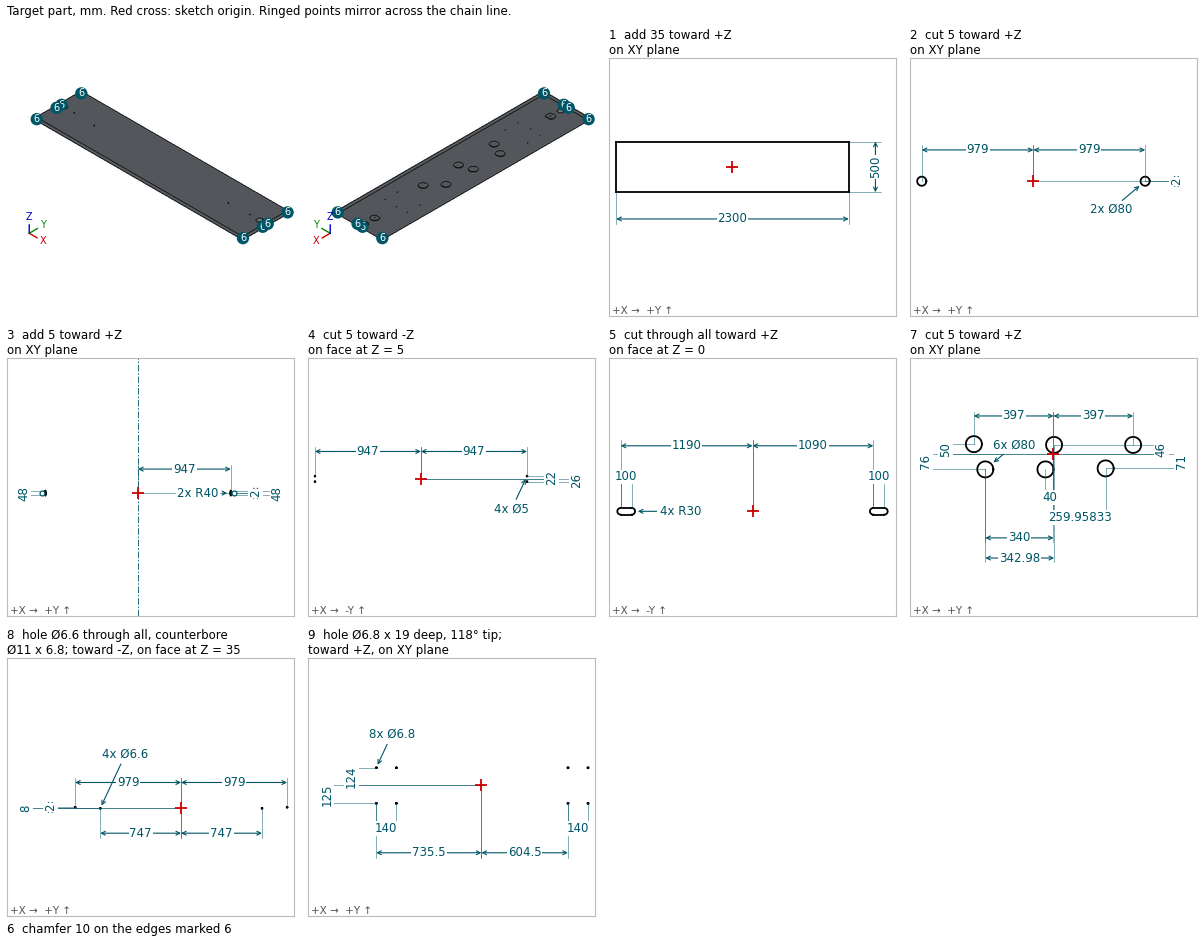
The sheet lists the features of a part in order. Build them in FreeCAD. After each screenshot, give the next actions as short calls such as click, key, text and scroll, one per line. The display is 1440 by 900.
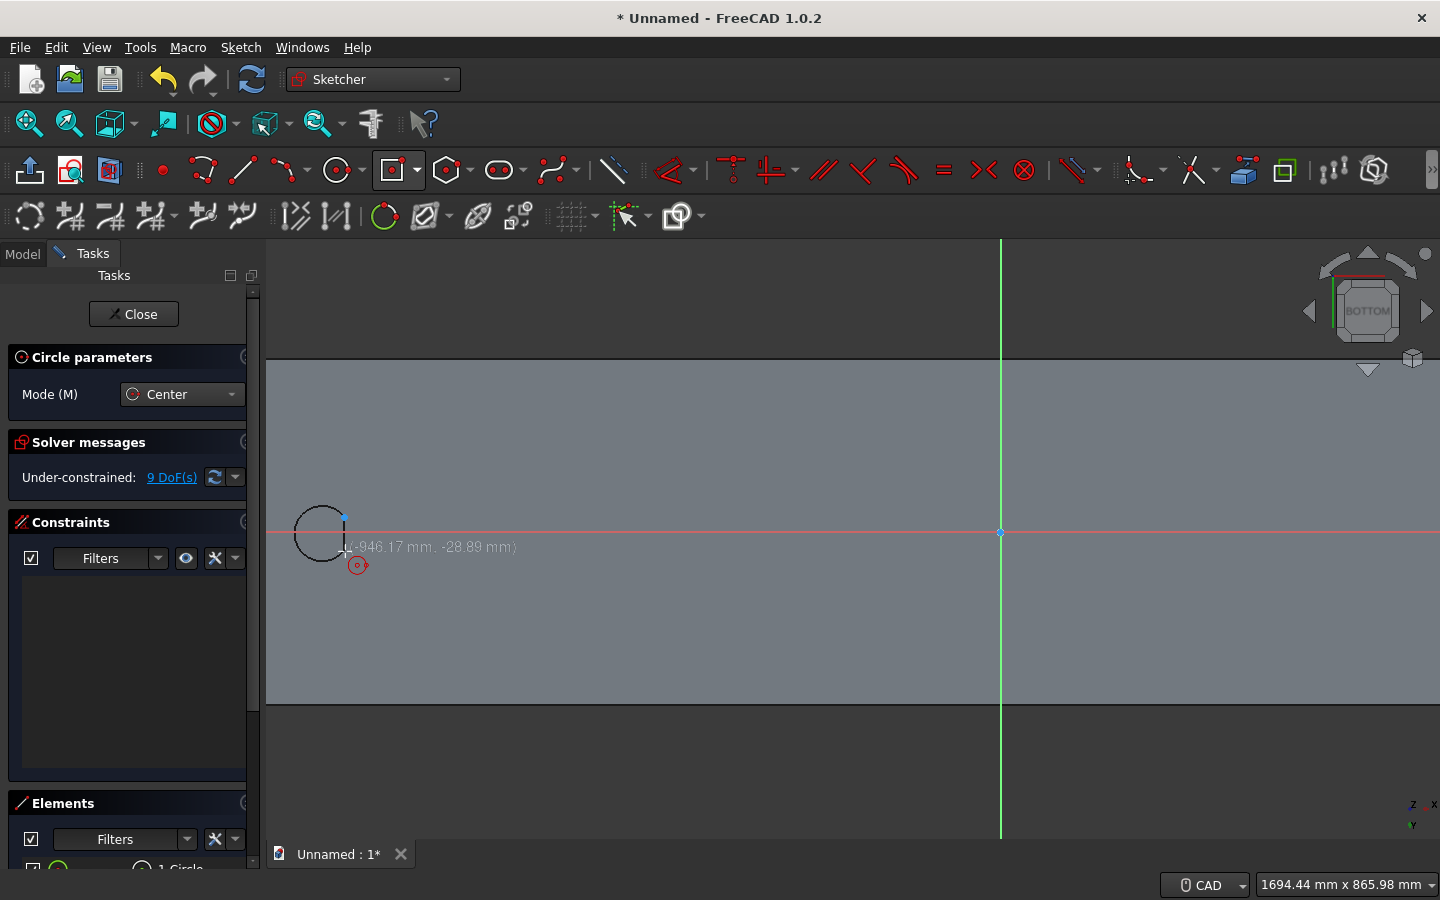
click(344, 550)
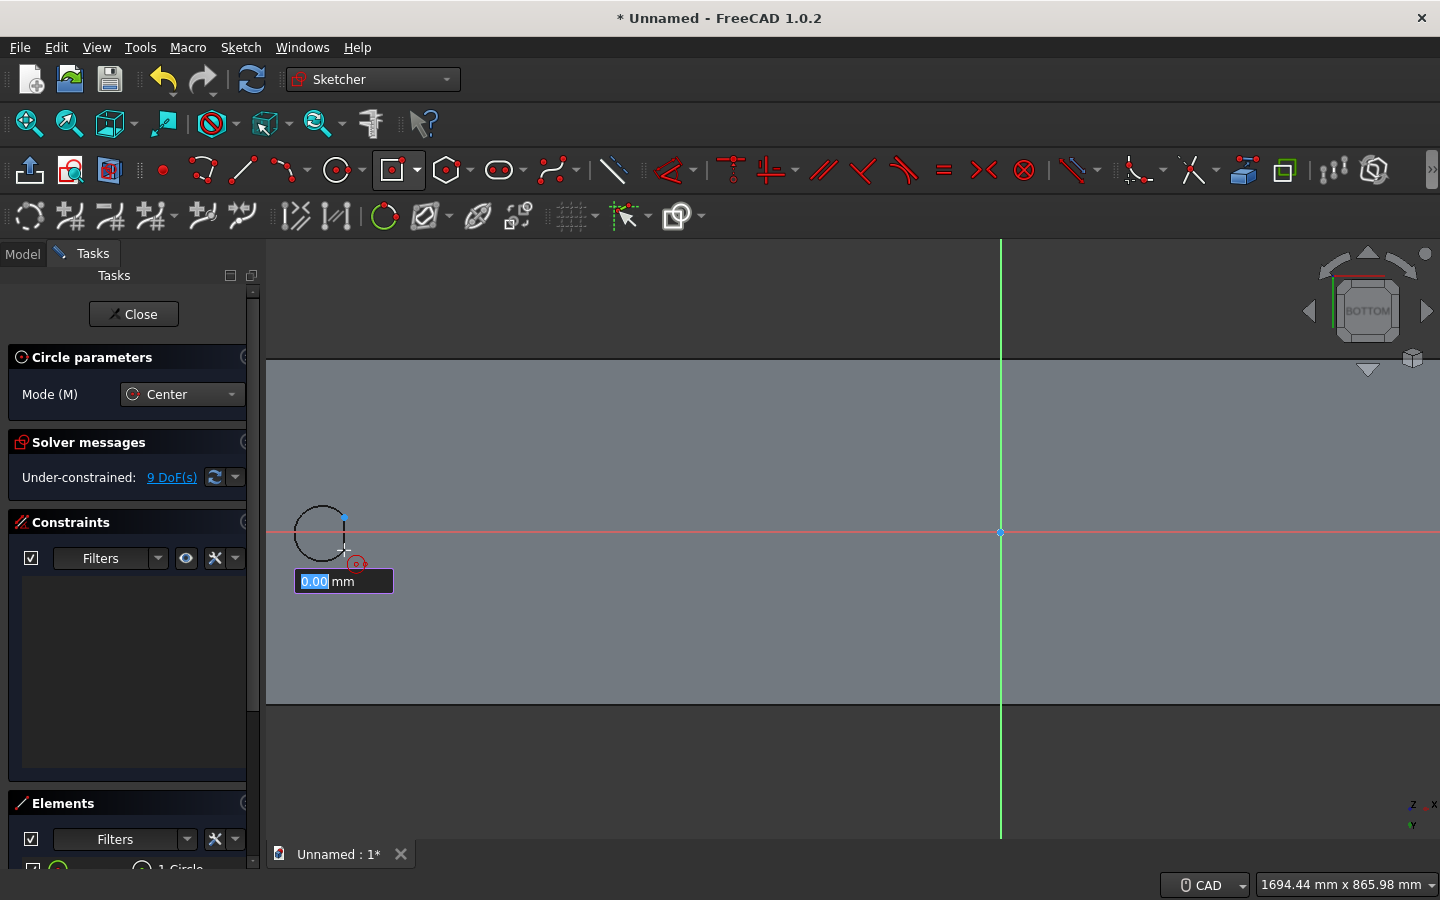
scroll(346, 549, up, 12)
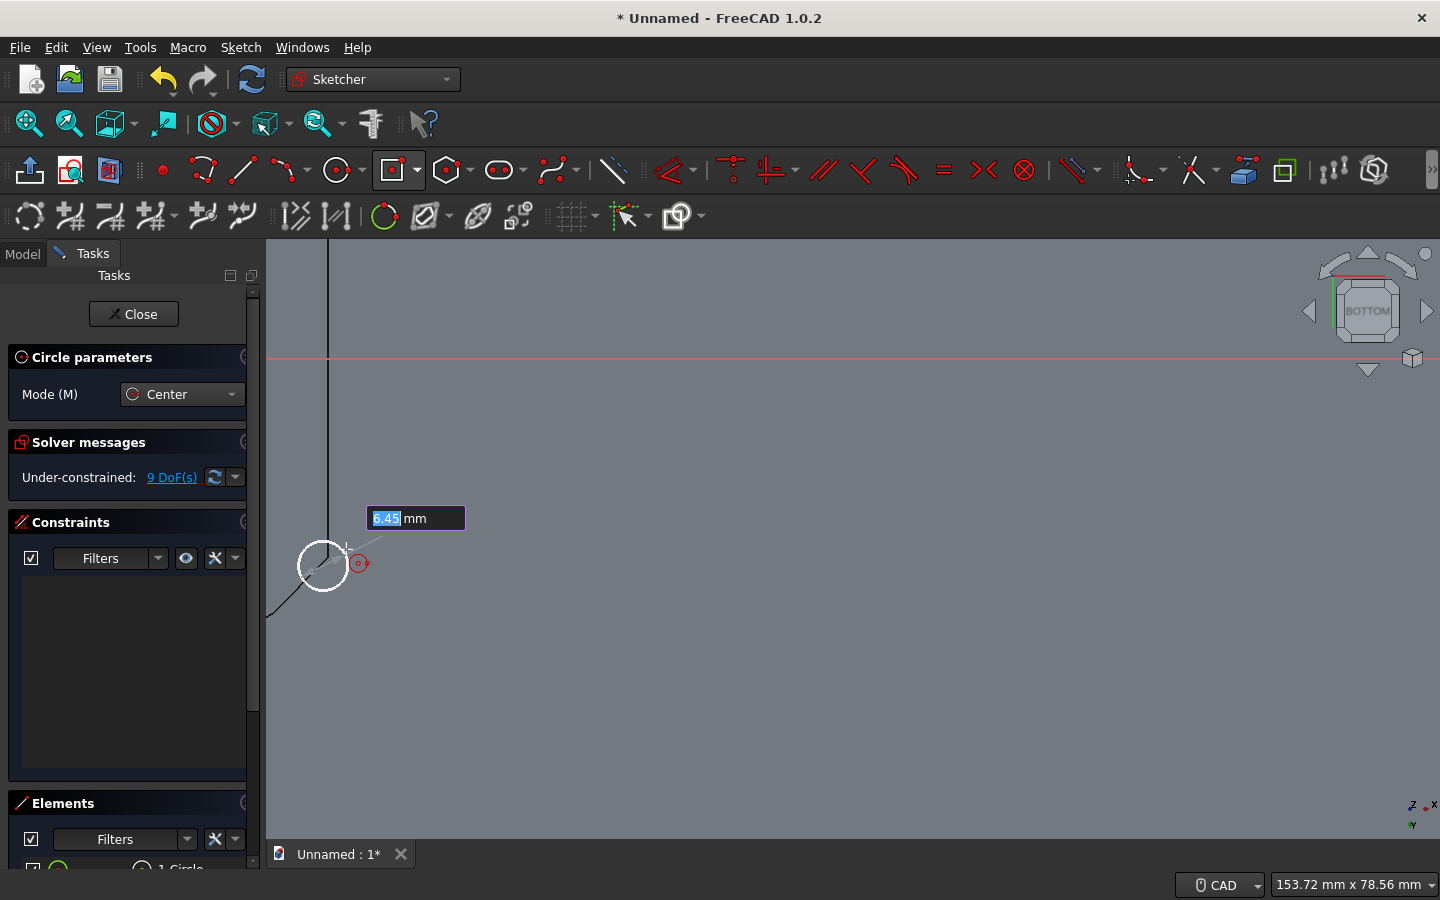
click(341, 544)
key(Escape)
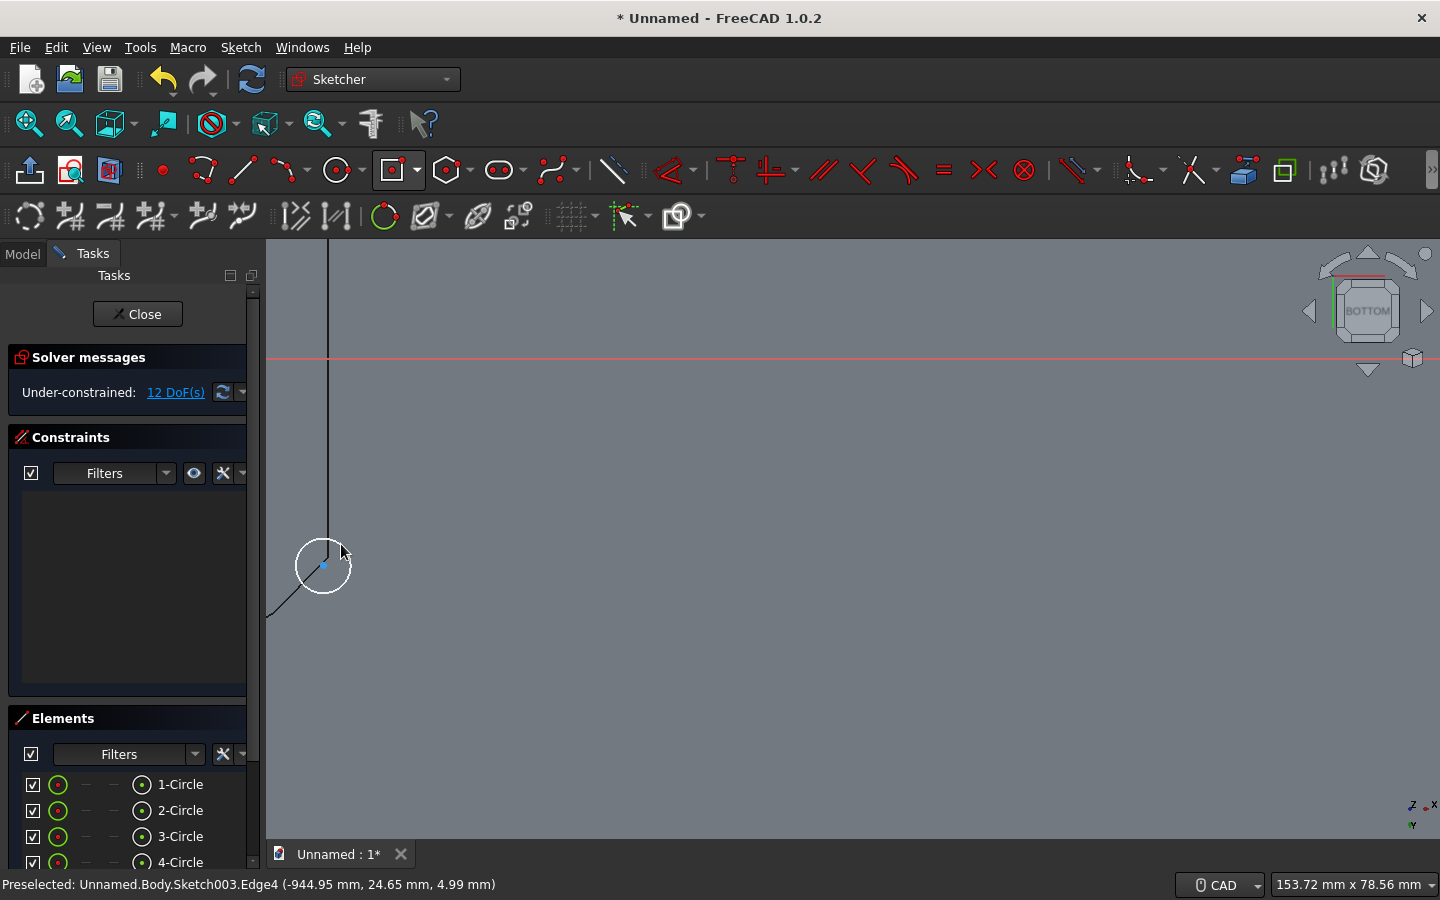
scroll(429, 548, down, 15)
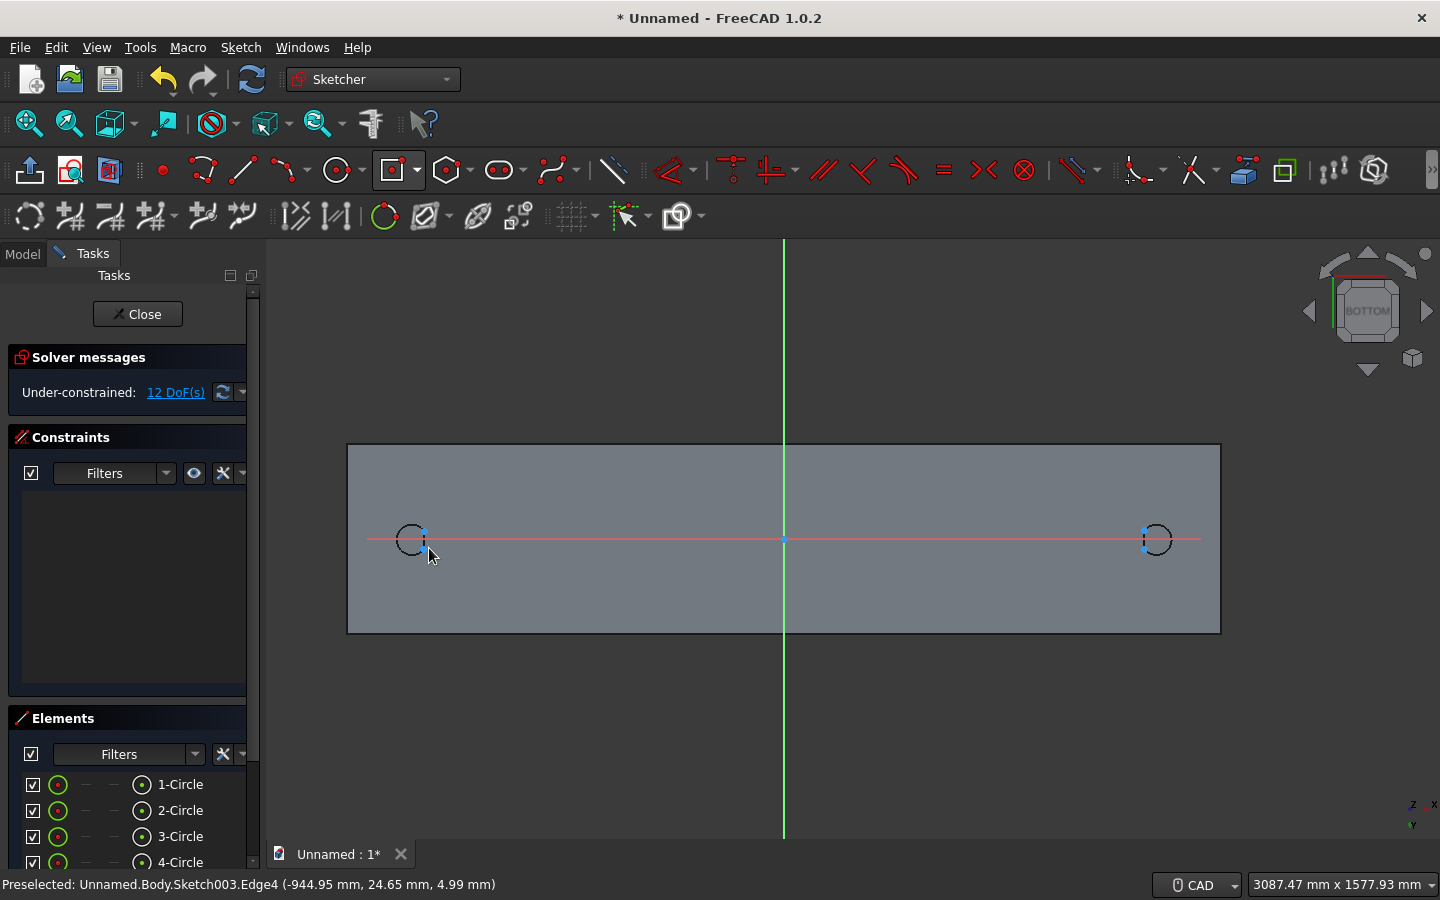
scroll(1145, 530, up, 13)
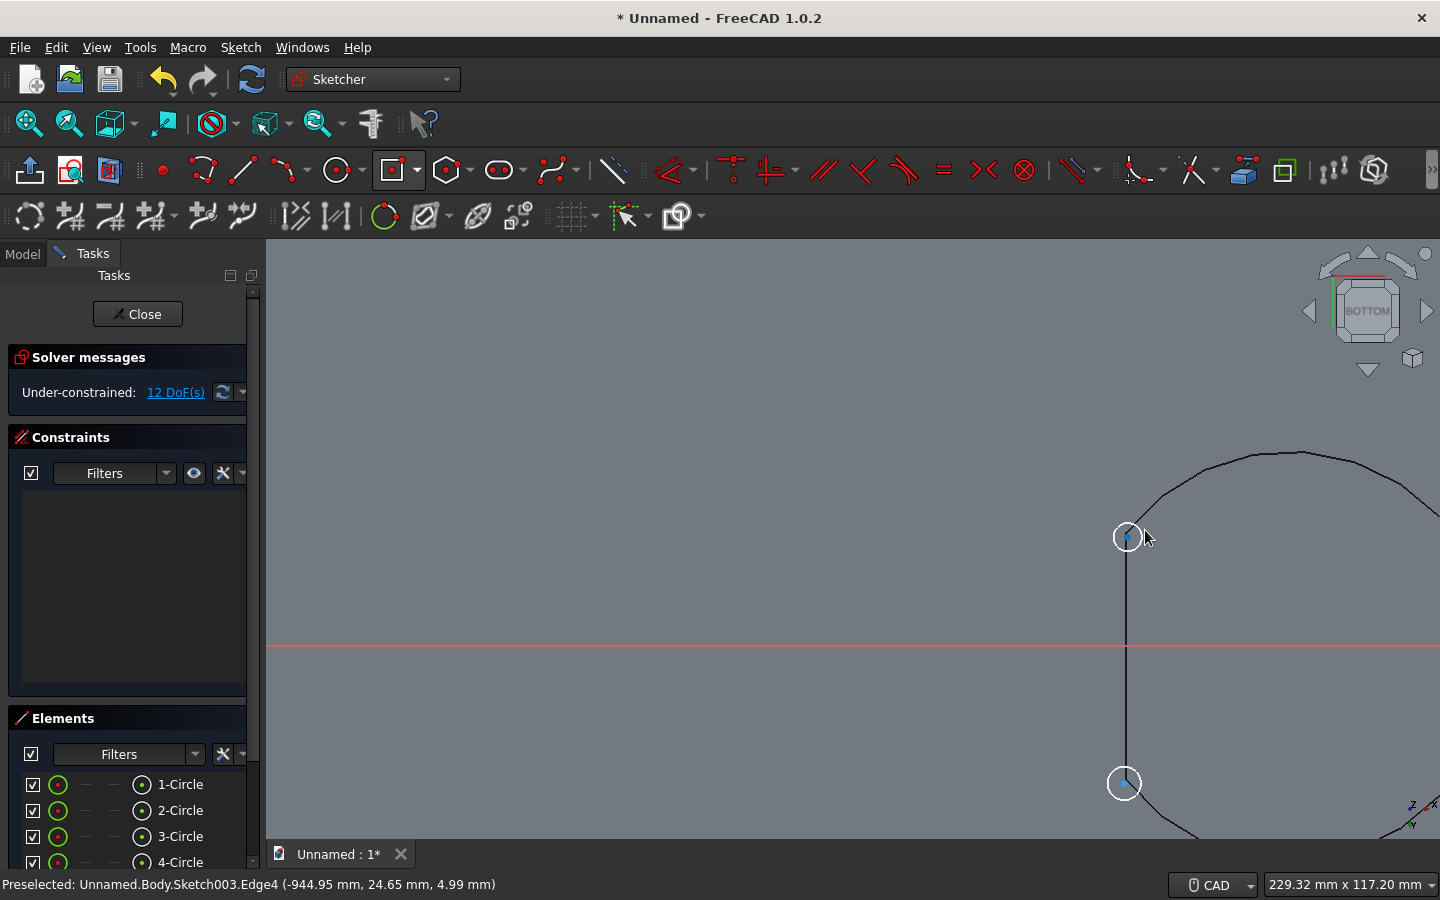
click(1138, 527)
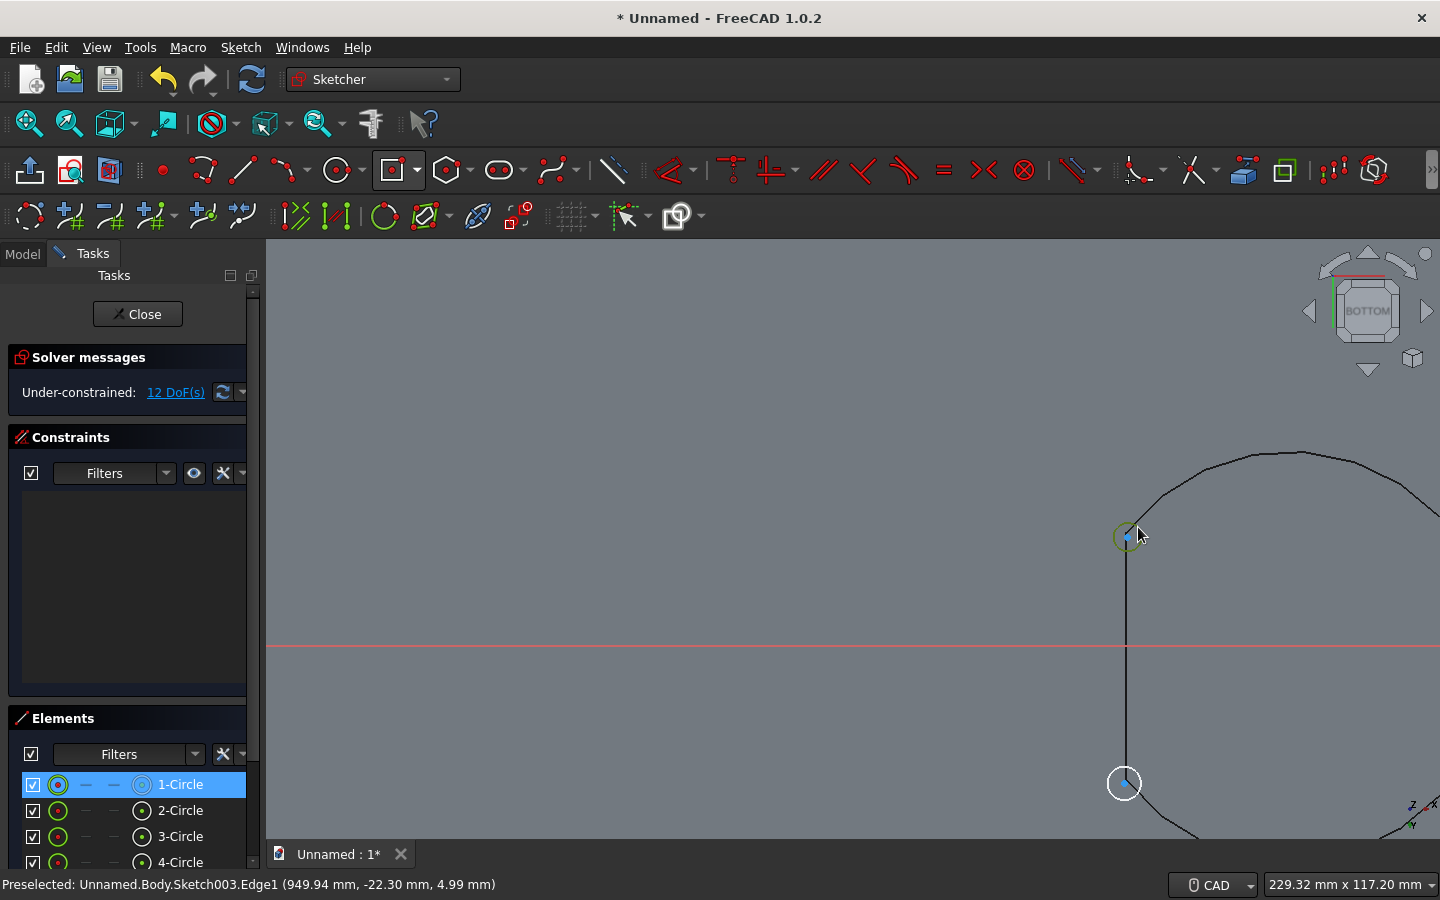
click(1136, 772)